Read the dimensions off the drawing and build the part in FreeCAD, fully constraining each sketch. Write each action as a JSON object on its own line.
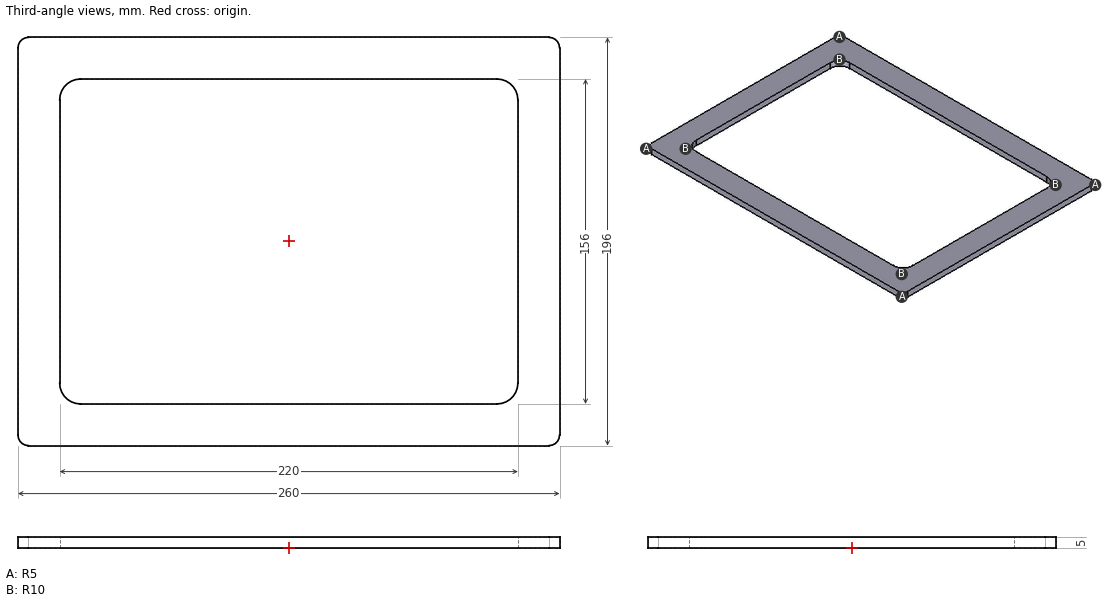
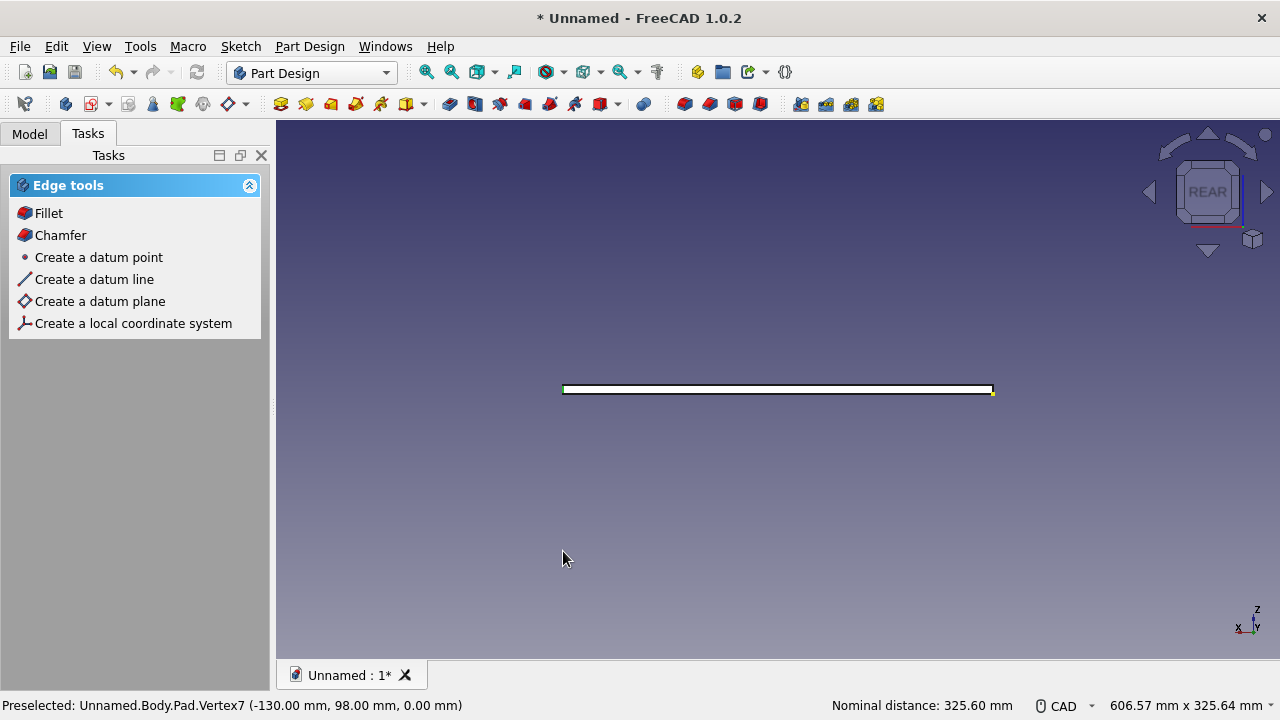
{"action": "left_click", "coordinate": [427, 72]}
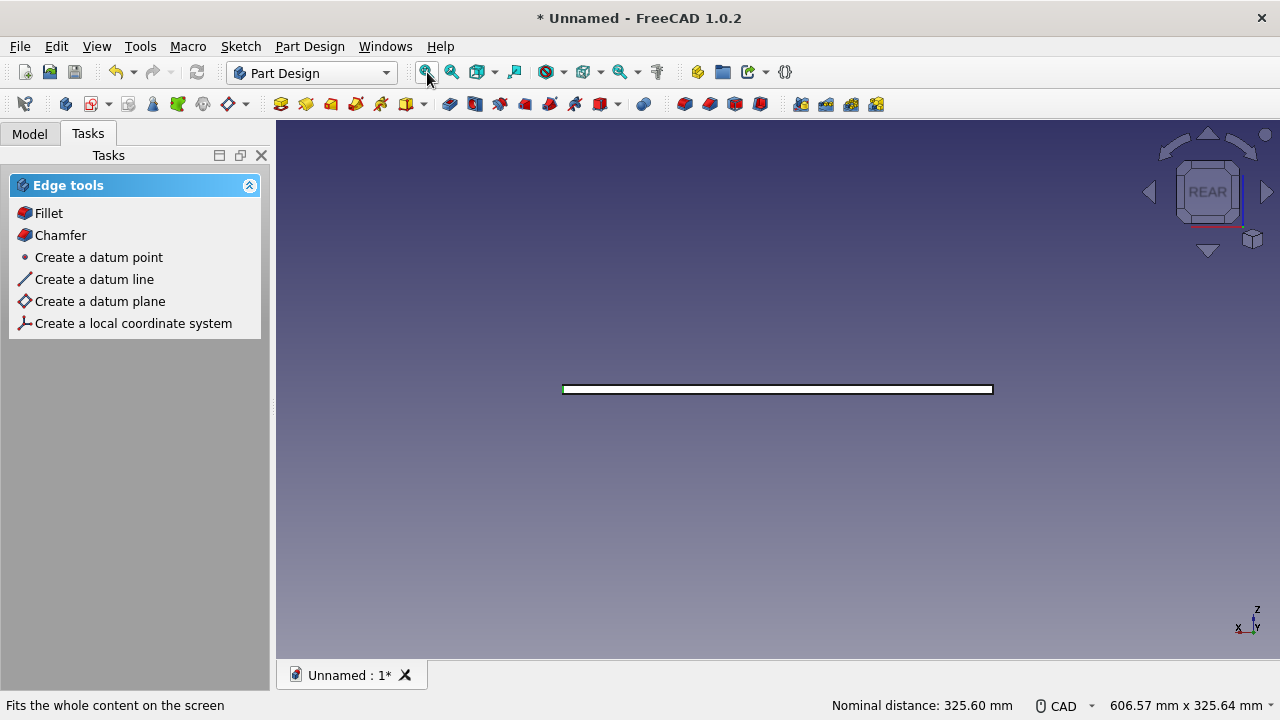
{"action": "scroll", "coordinate": [993, 389], "scroll_direction": "up", "scroll_amount": 8}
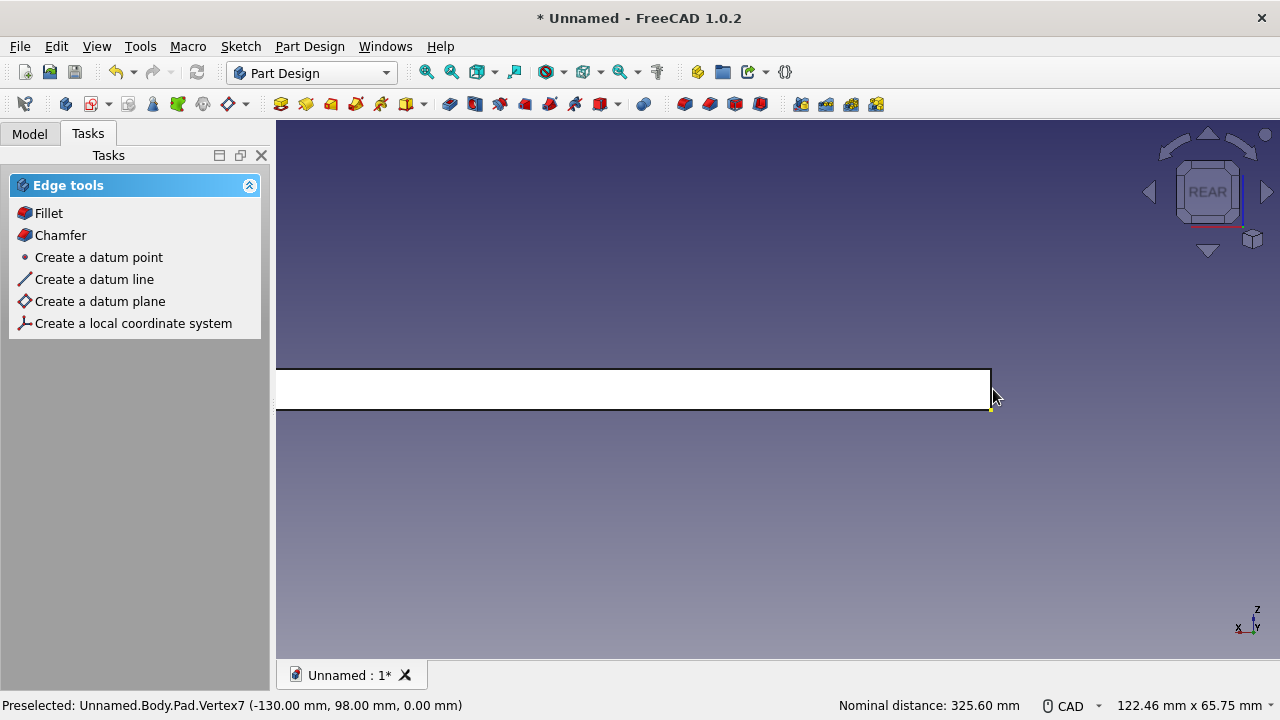
{"action": "left_click", "coordinate": [991, 389], "text": "ctrl"}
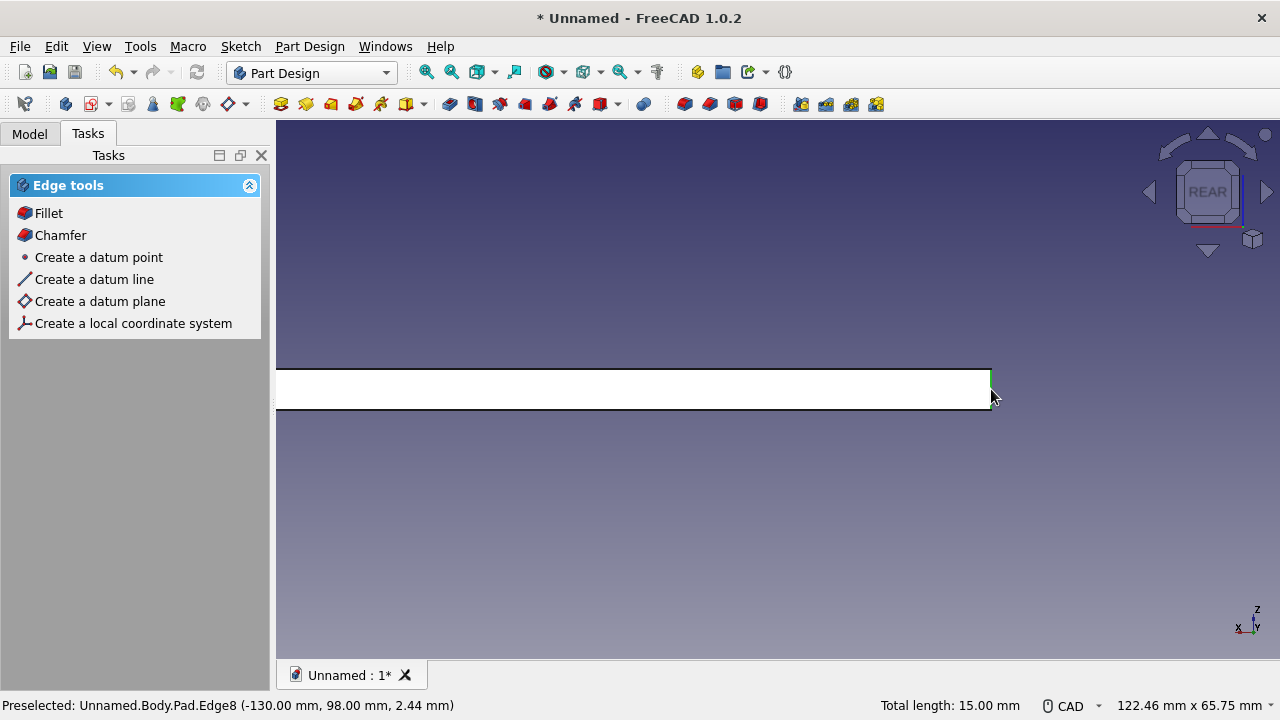
{"action": "left_click", "coordinate": [427, 72]}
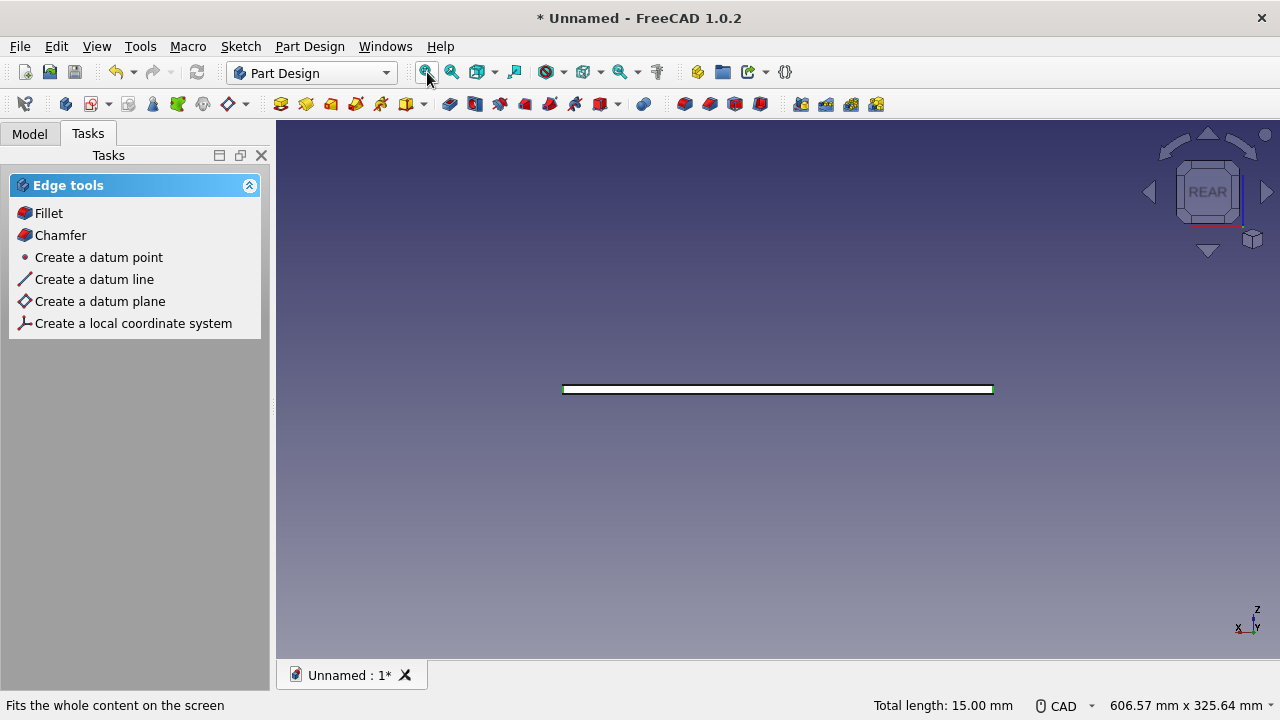
{"action": "key", "text": "6"}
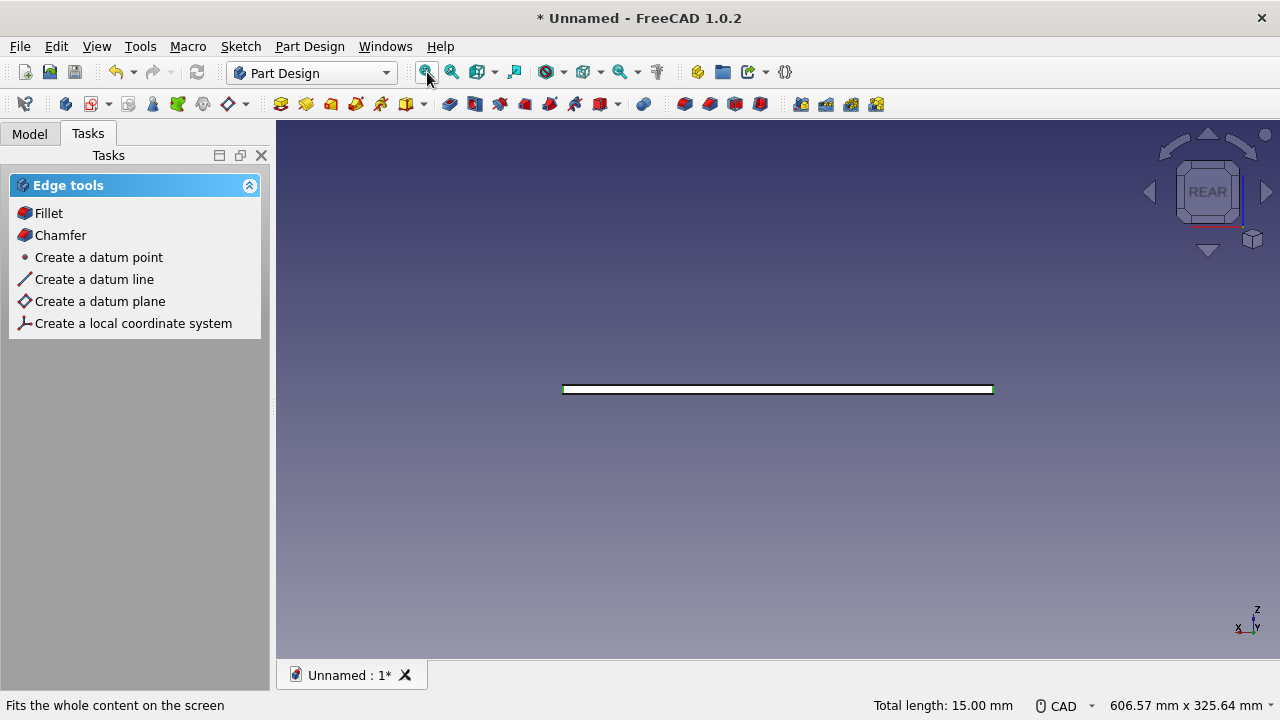
{"action": "left_click", "coordinate": [427, 72]}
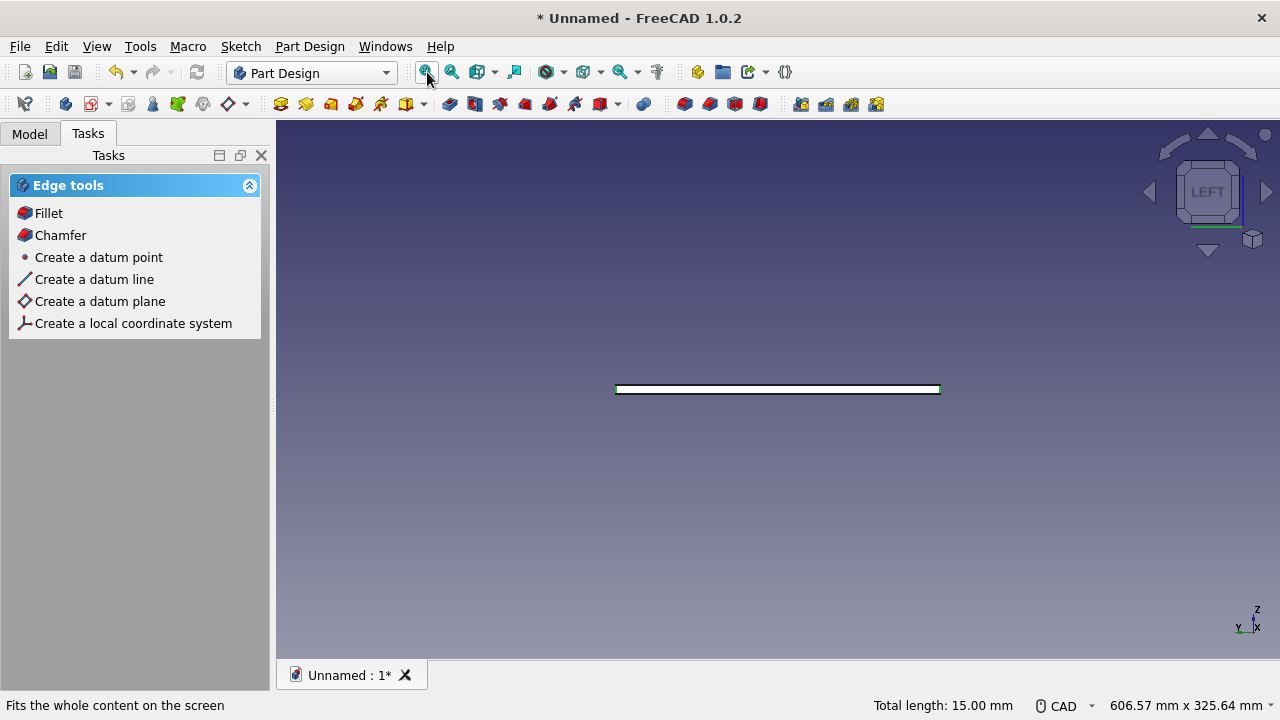
{"action": "scroll", "coordinate": [940, 388], "scroll_direction": "up", "scroll_amount": 8}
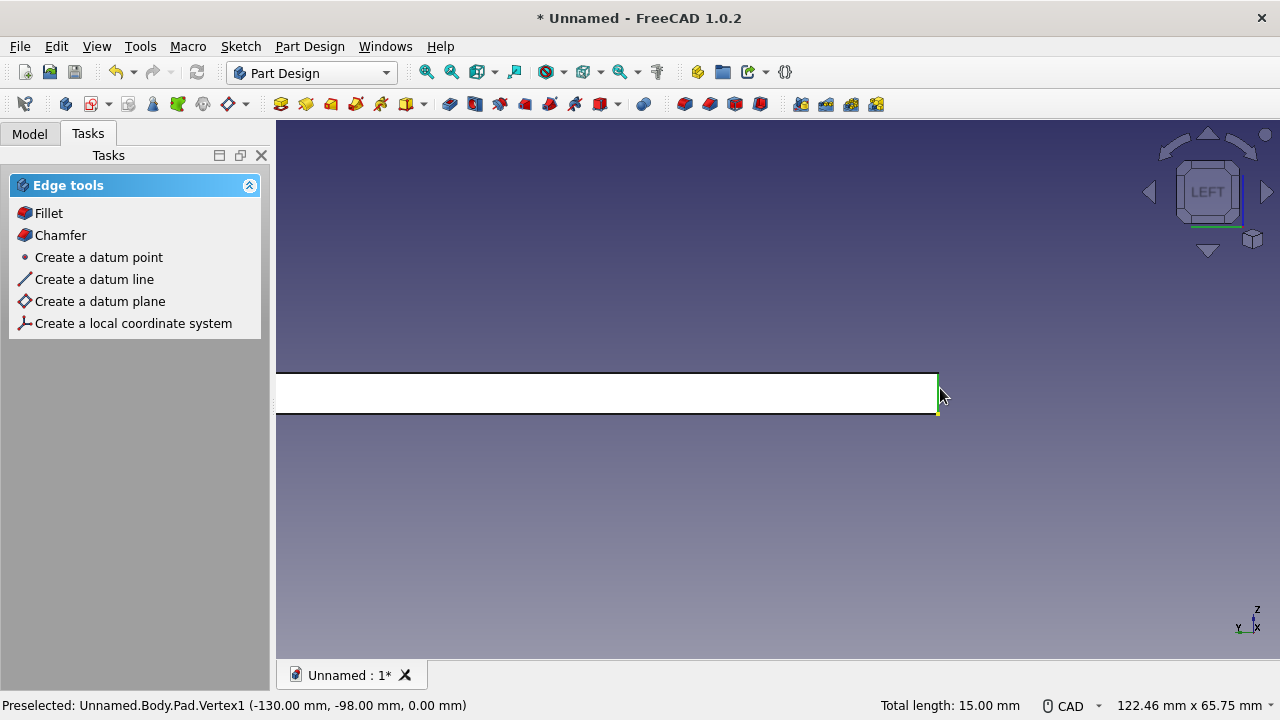
{"action": "left_click", "coordinate": [427, 72]}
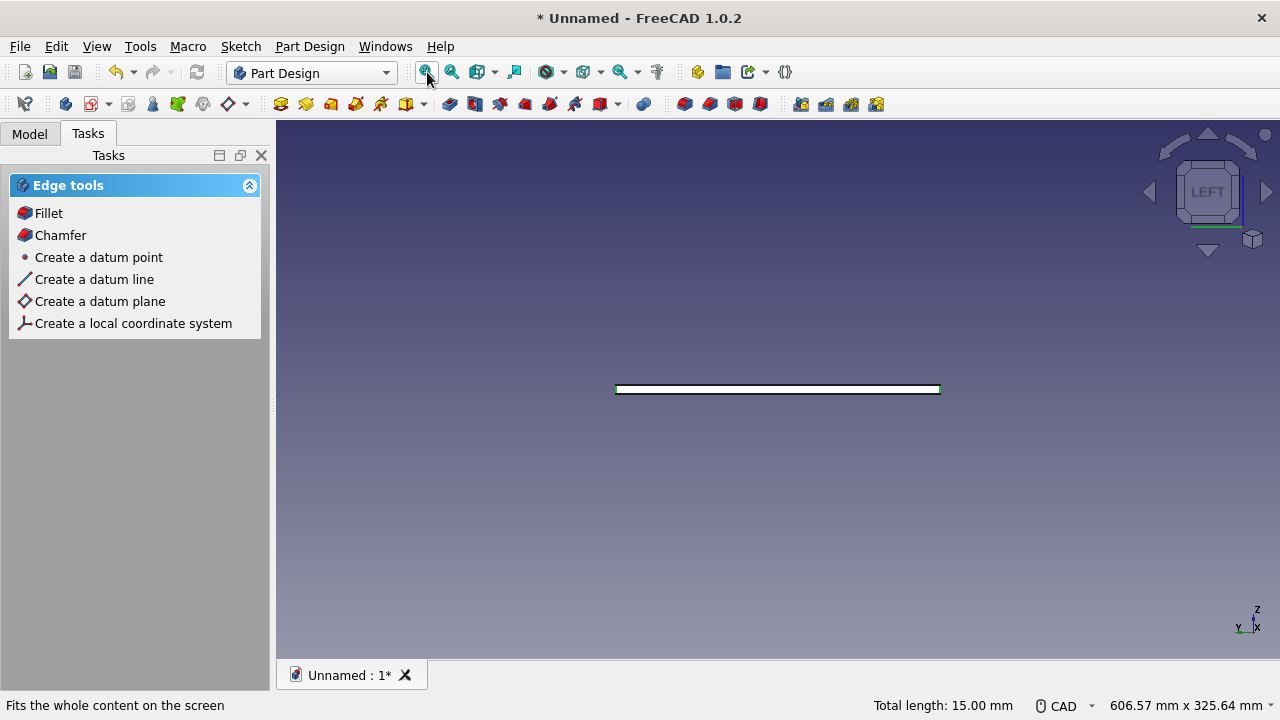
{"action": "key", "text": "v 3"}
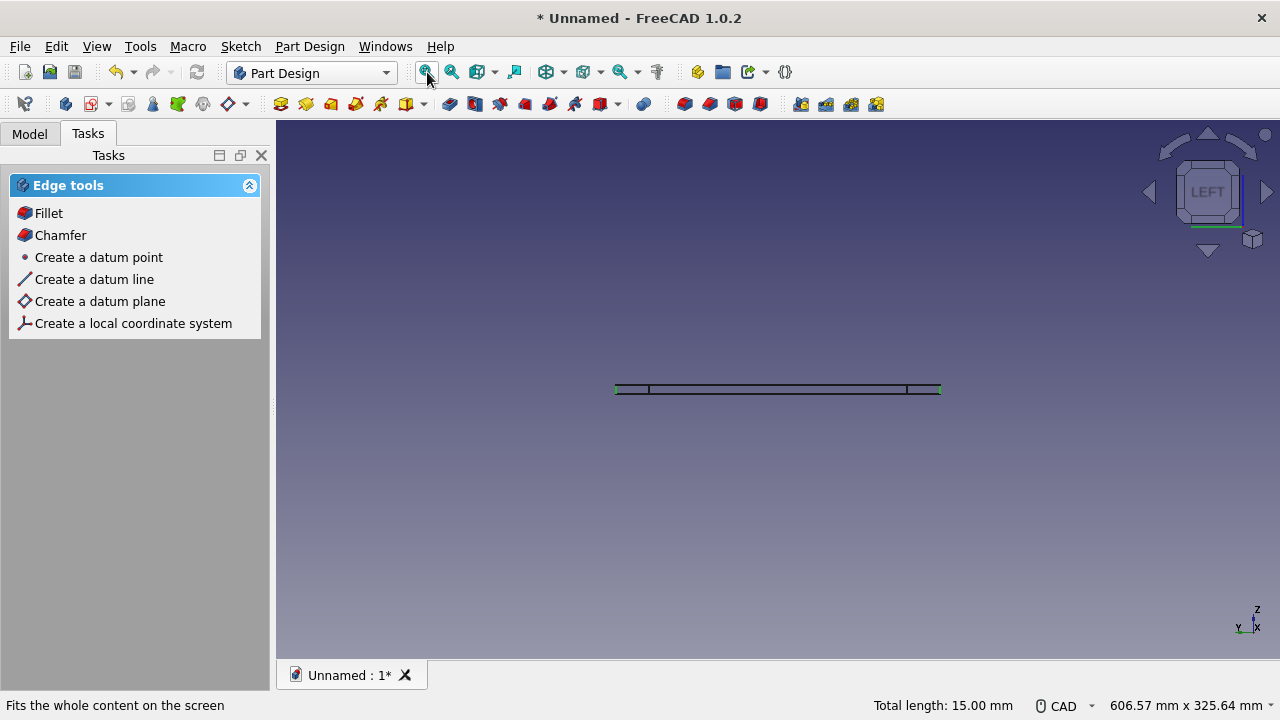
{"action": "key", "text": "0"}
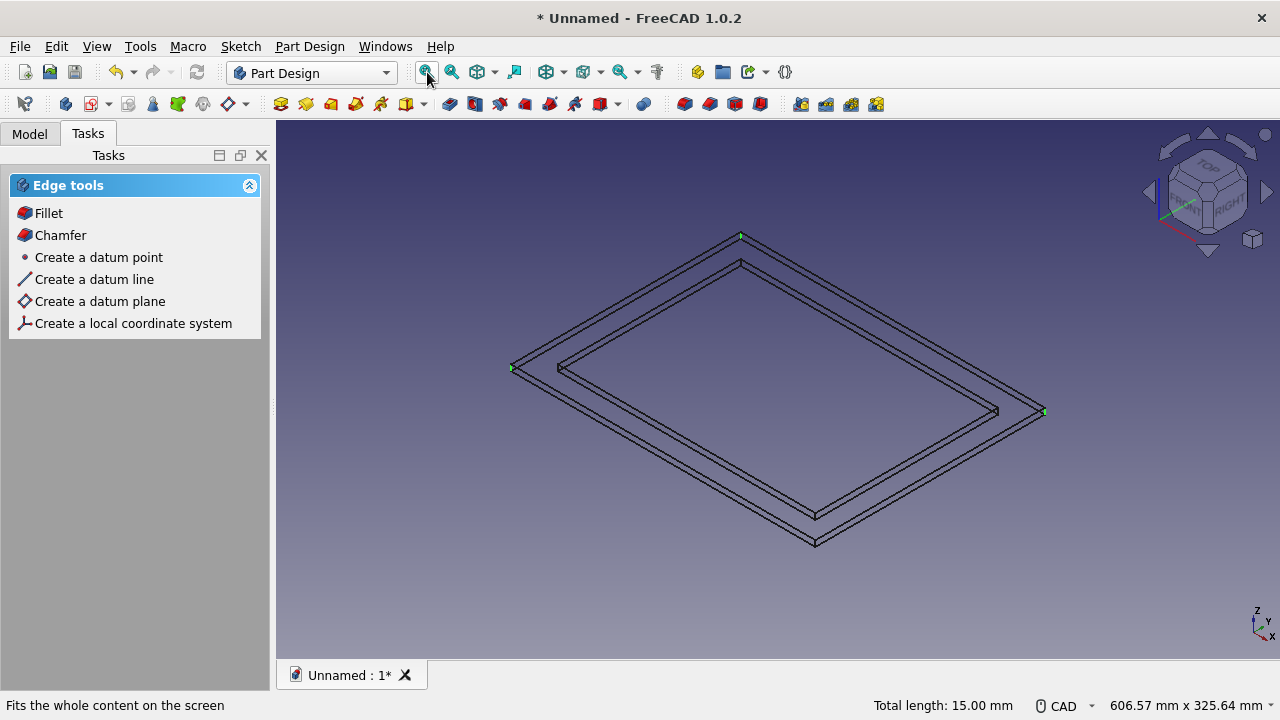
{"action": "scroll", "coordinate": [815, 543], "scroll_direction": "up", "scroll_amount": 8}